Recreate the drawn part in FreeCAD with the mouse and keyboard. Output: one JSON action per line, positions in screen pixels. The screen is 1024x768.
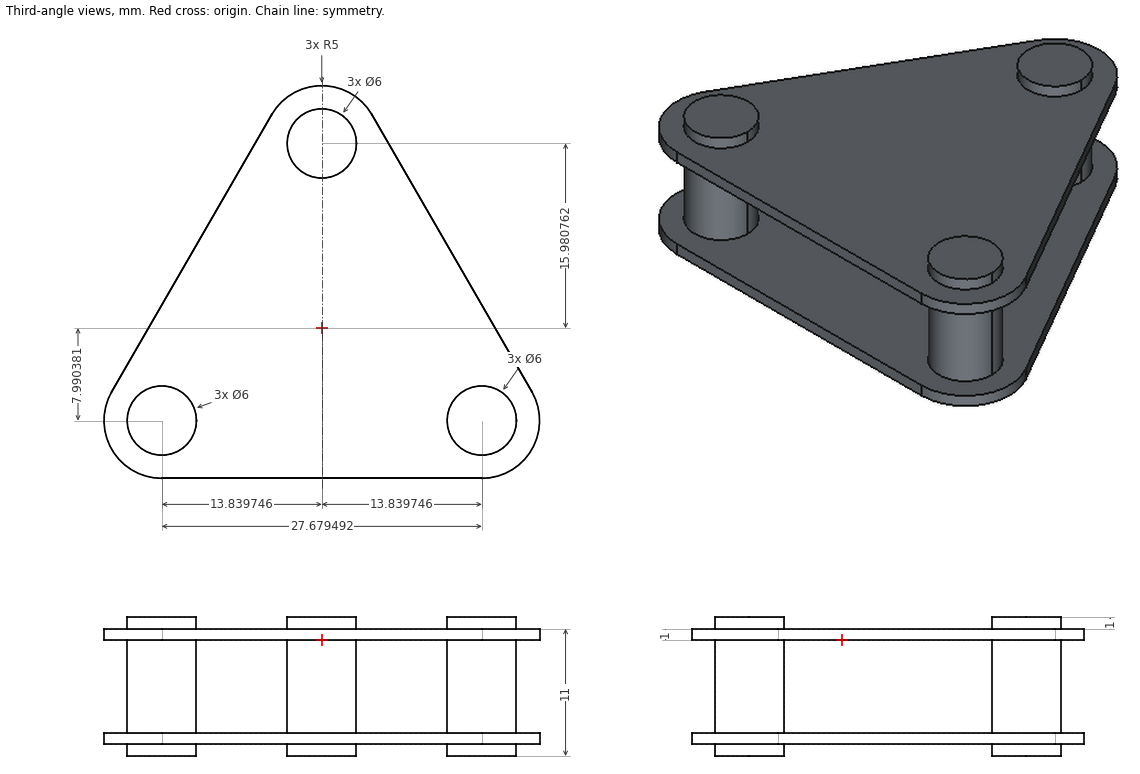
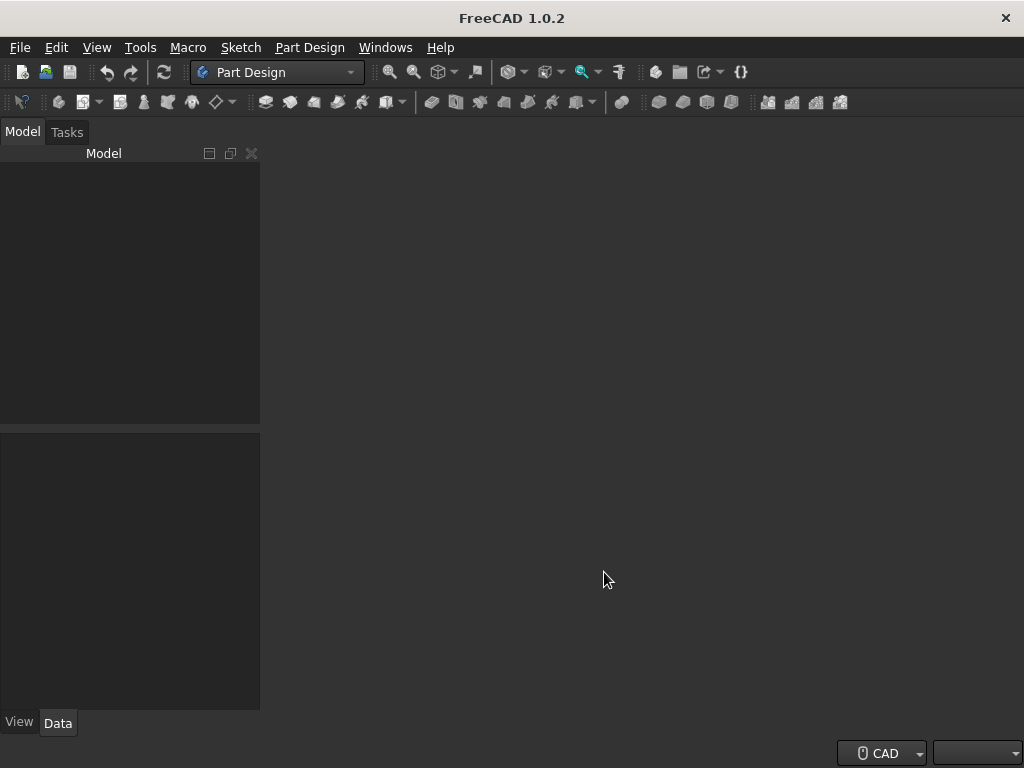
{"action": "left_click", "coordinate": [22, 72]}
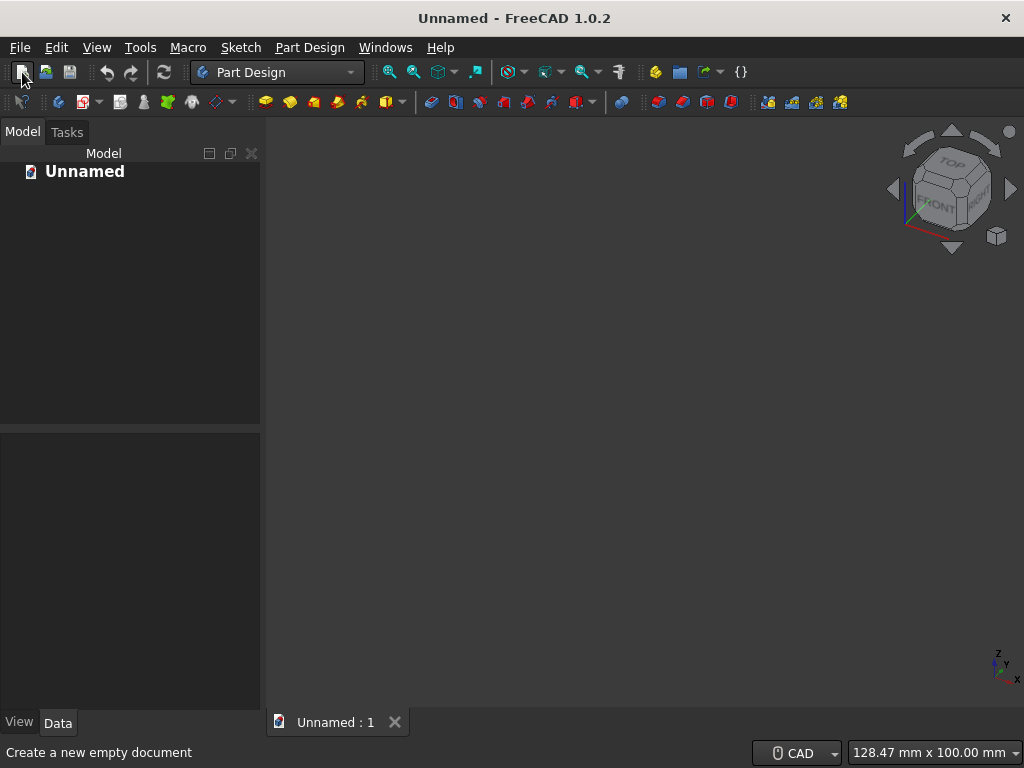
{"action": "left_click", "coordinate": [84, 102]}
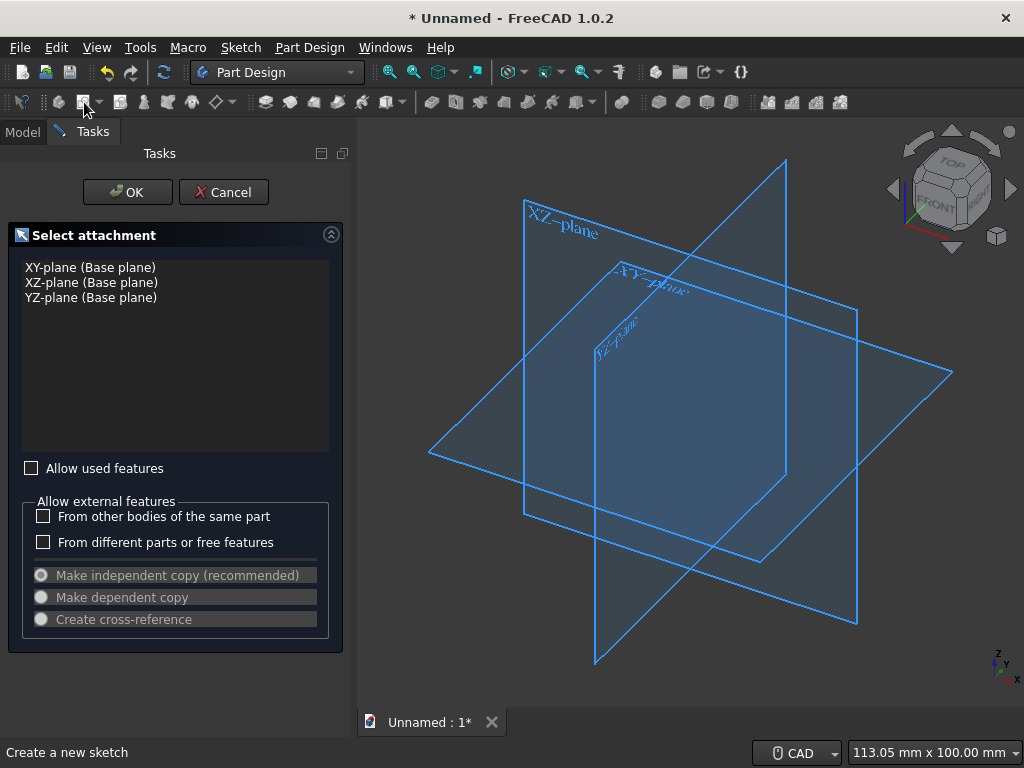
{"action": "left_click", "coordinate": [82, 268]}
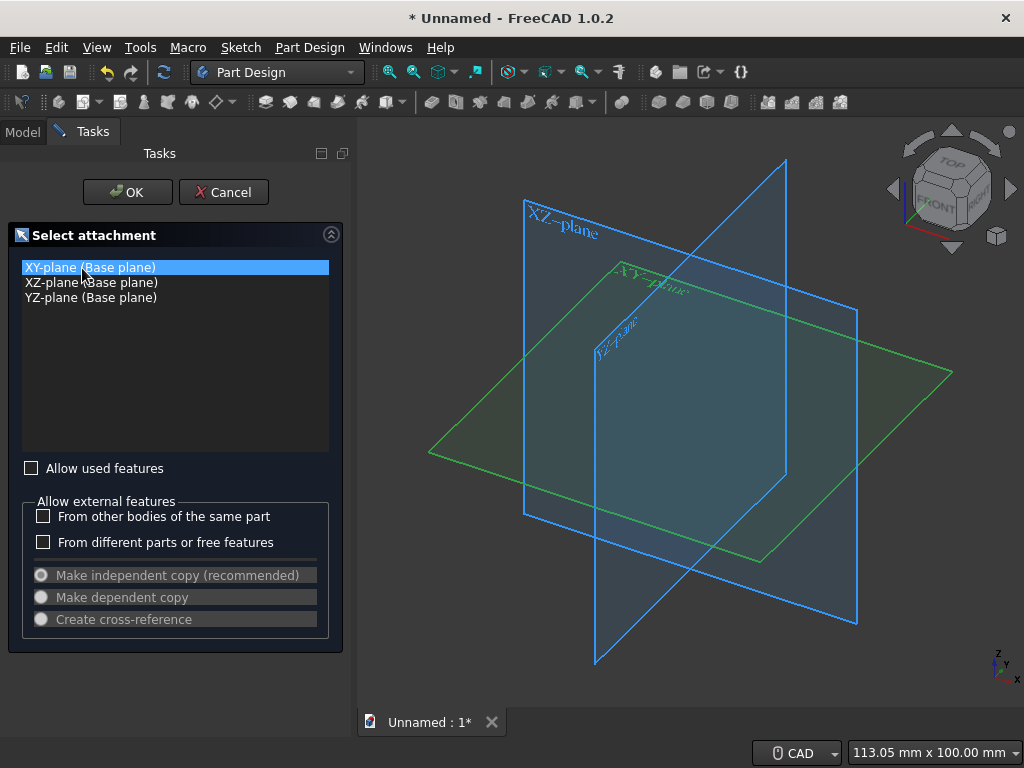
{"action": "left_click", "coordinate": [128, 192]}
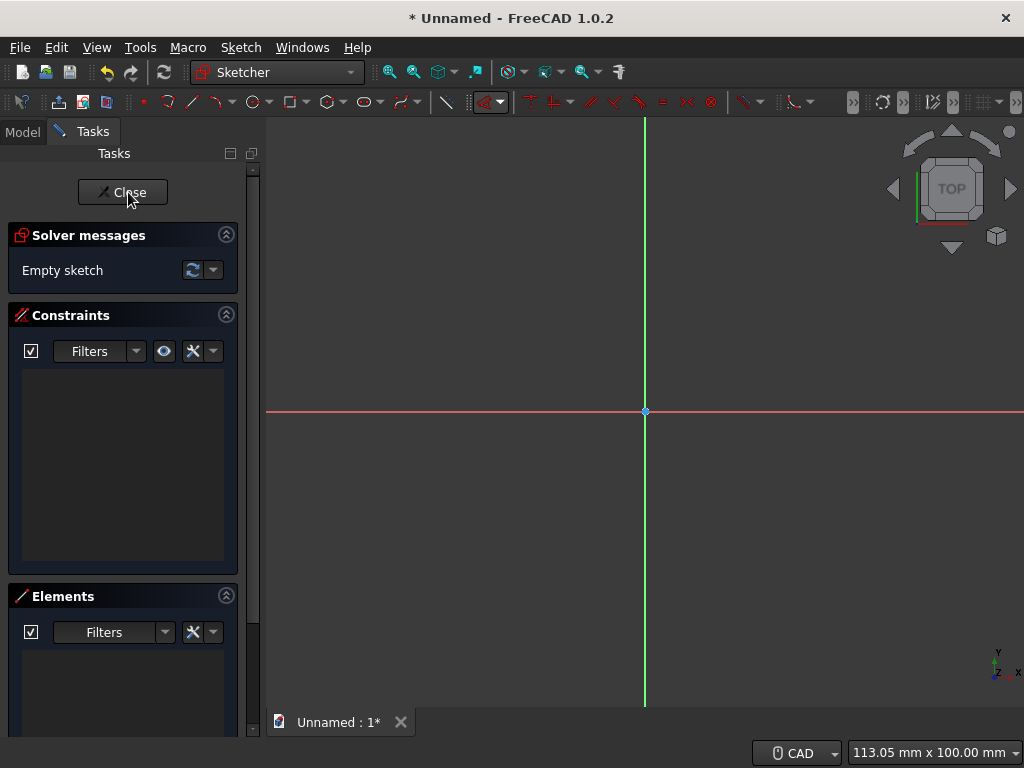
{"action": "scroll", "coordinate": [728, 360], "scroll_direction": "up", "scroll_amount": 3}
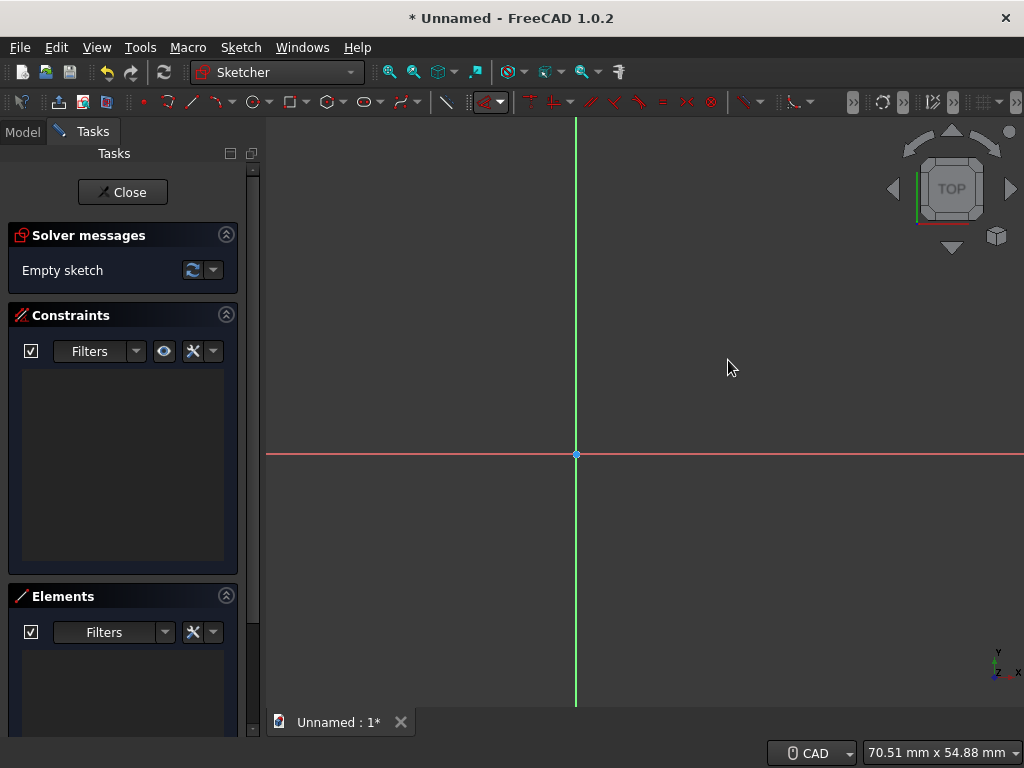
{"action": "left_click", "coordinate": [192, 102]}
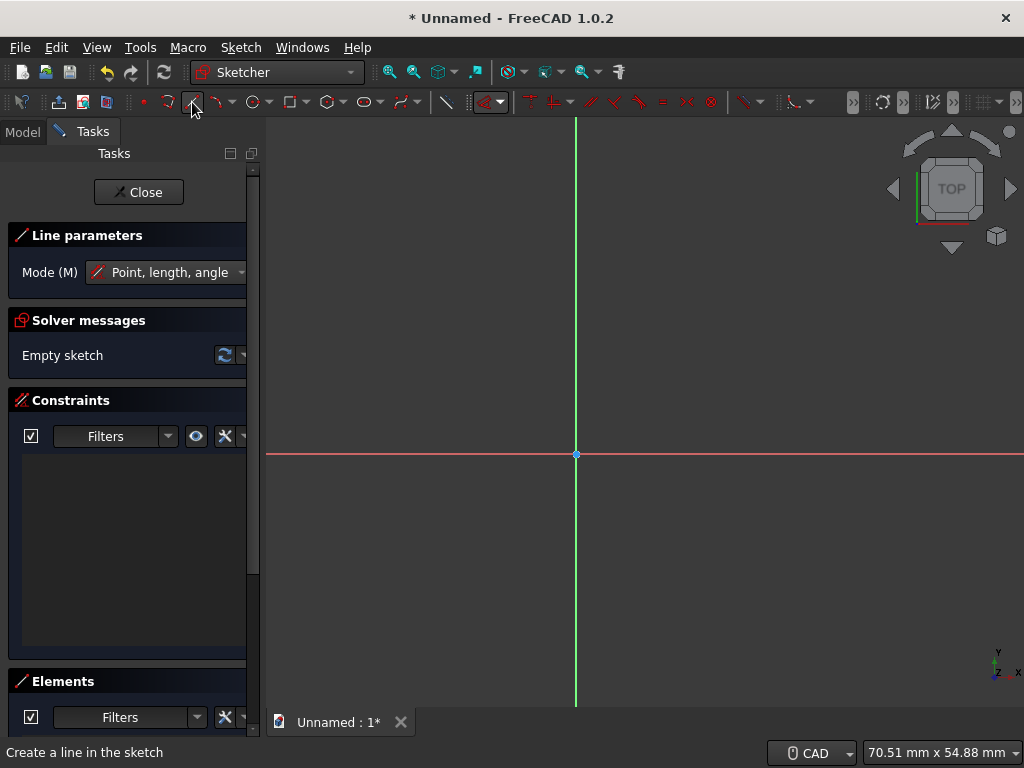
{"action": "left_click", "coordinate": [772, 513]}
{"action": "left_click", "coordinate": [623, 256]}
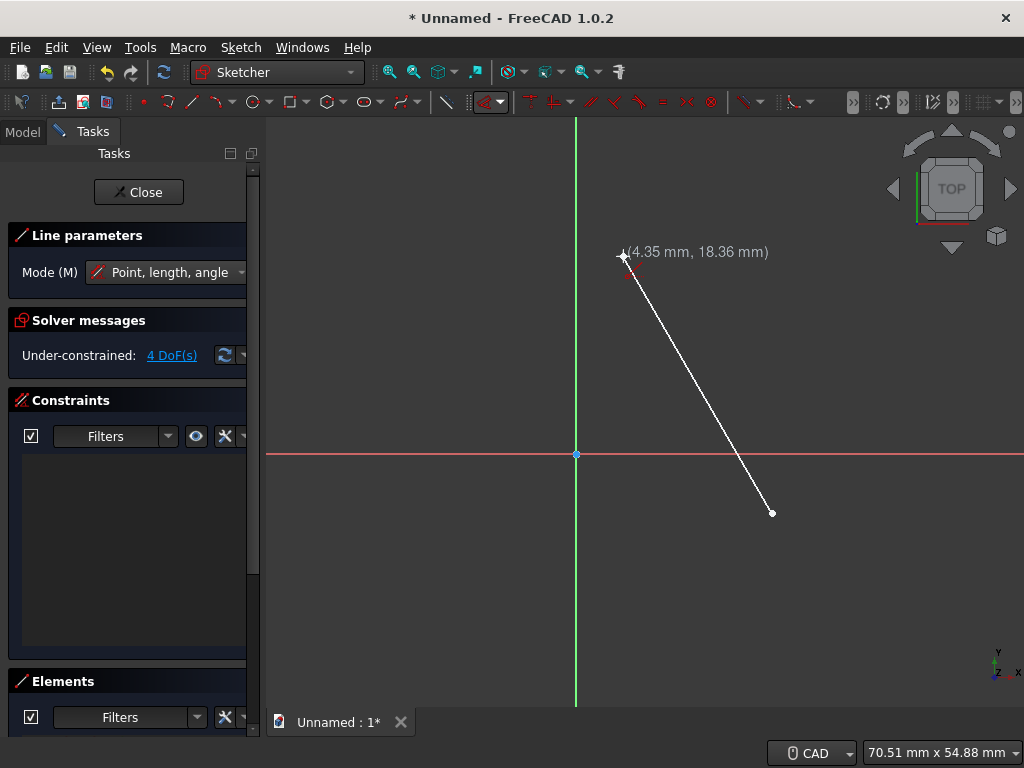
{"action": "left_click", "coordinate": [530, 256]}
{"action": "left_click", "coordinate": [381, 513]}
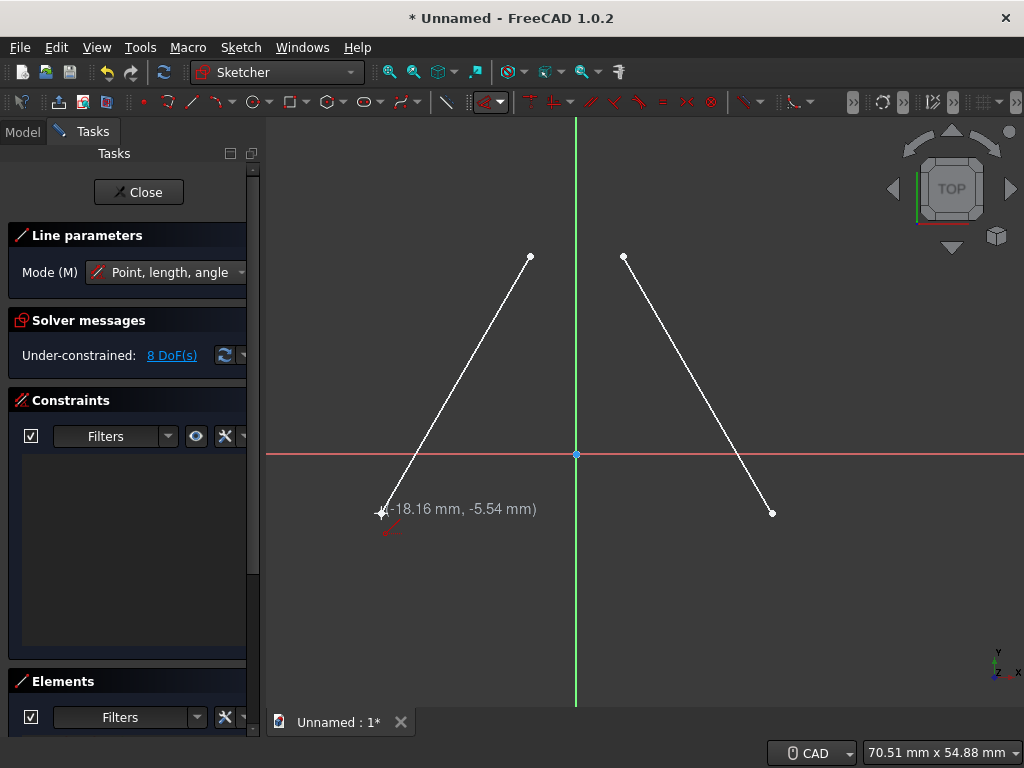
{"action": "left_click", "coordinate": [427, 594]}
{"action": "left_click", "coordinate": [725, 594]}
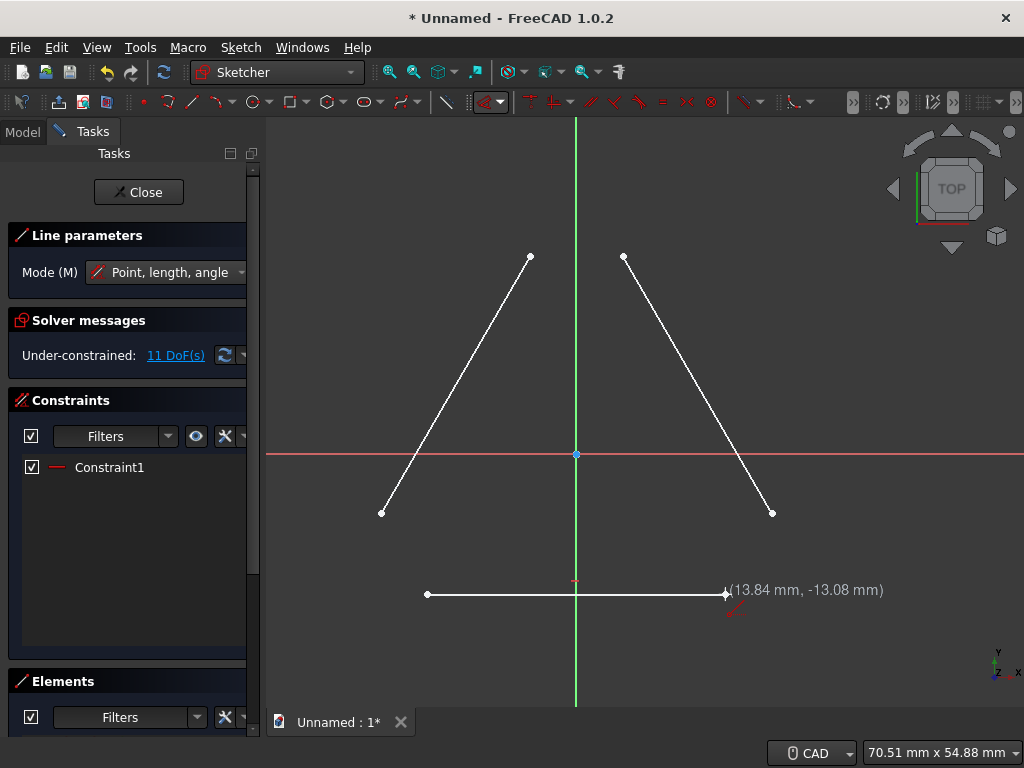
{"action": "left_click", "coordinate": [216, 102]}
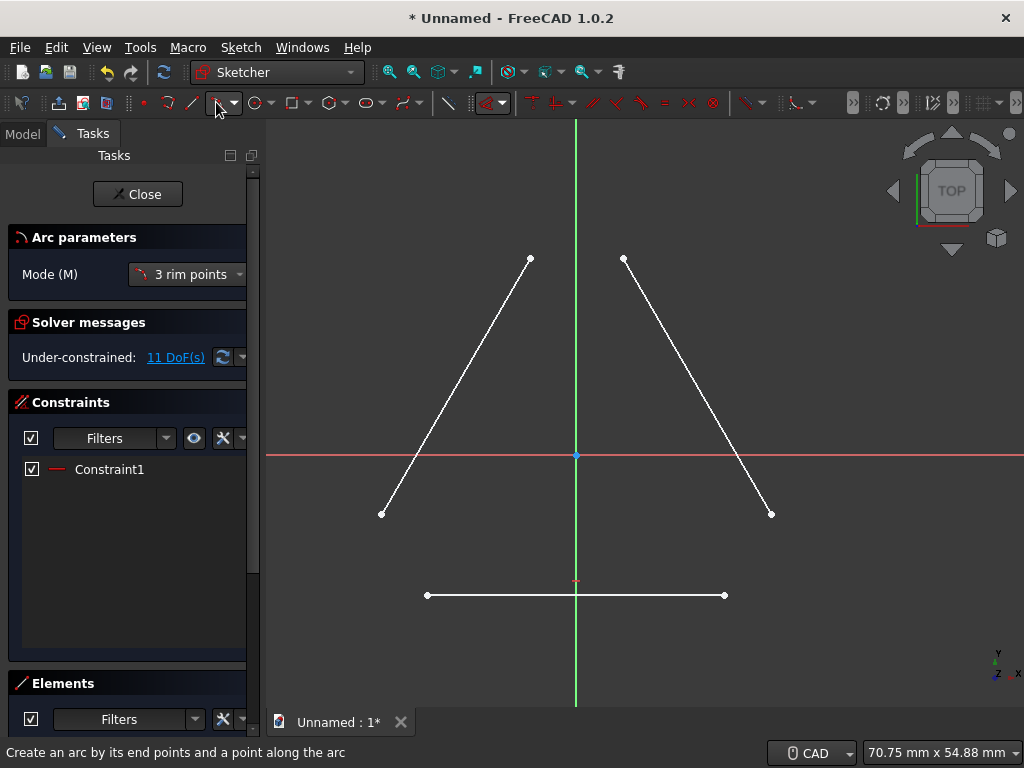
{"action": "left_click", "coordinate": [623, 259]}
{"action": "left_click", "coordinate": [530, 259]}
{"action": "left_click", "coordinate": [598, 235]}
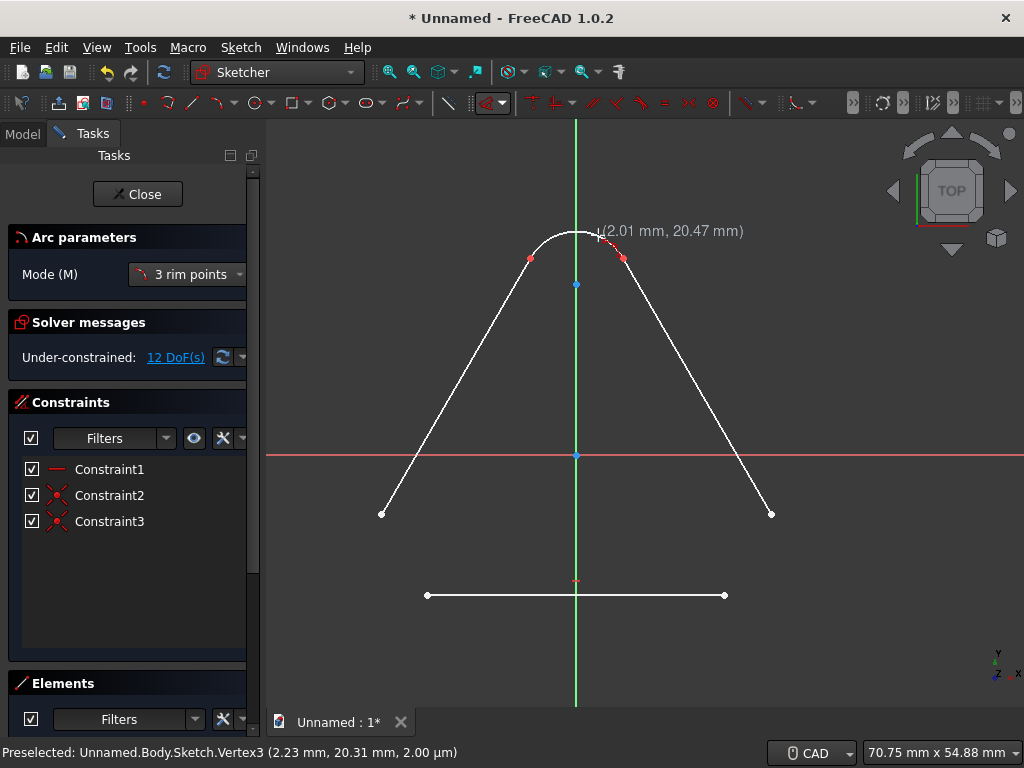
{"action": "left_click", "coordinate": [382, 515]}
{"action": "left_click", "coordinate": [428, 595]}
{"action": "left_click", "coordinate": [382, 568]}